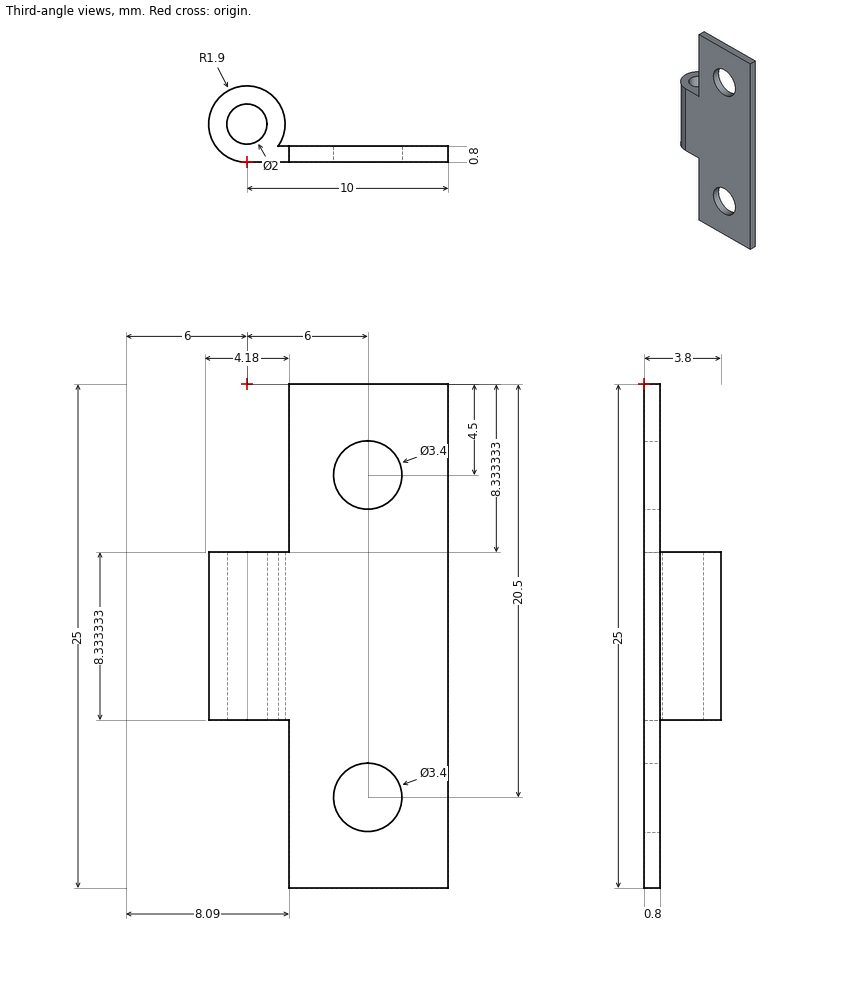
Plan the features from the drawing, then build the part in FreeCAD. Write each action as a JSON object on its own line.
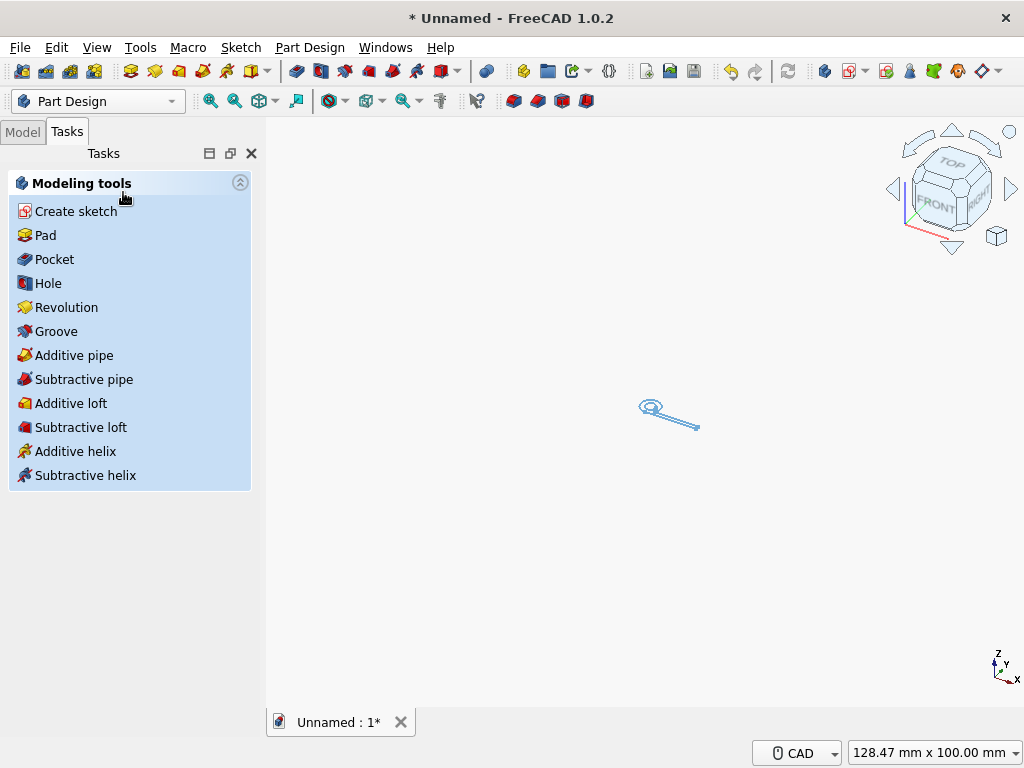
{"action": "left_click", "coordinate": [132, 72]}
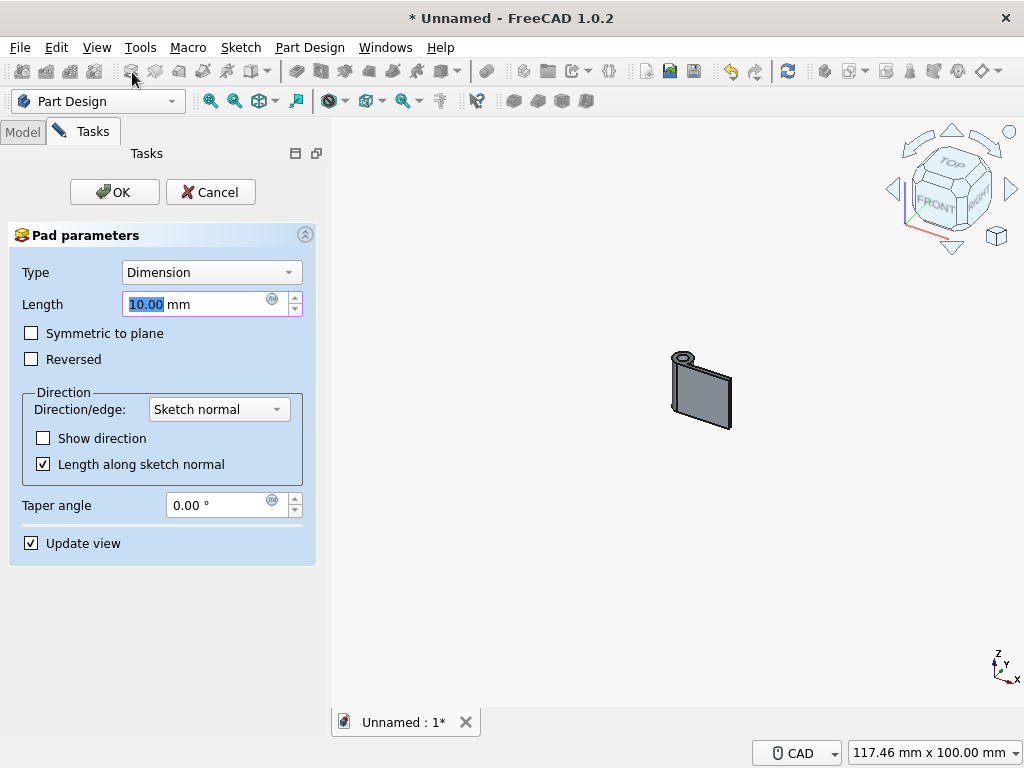
{"action": "type", "text": "25"}
{"action": "key", "text": "Tab"}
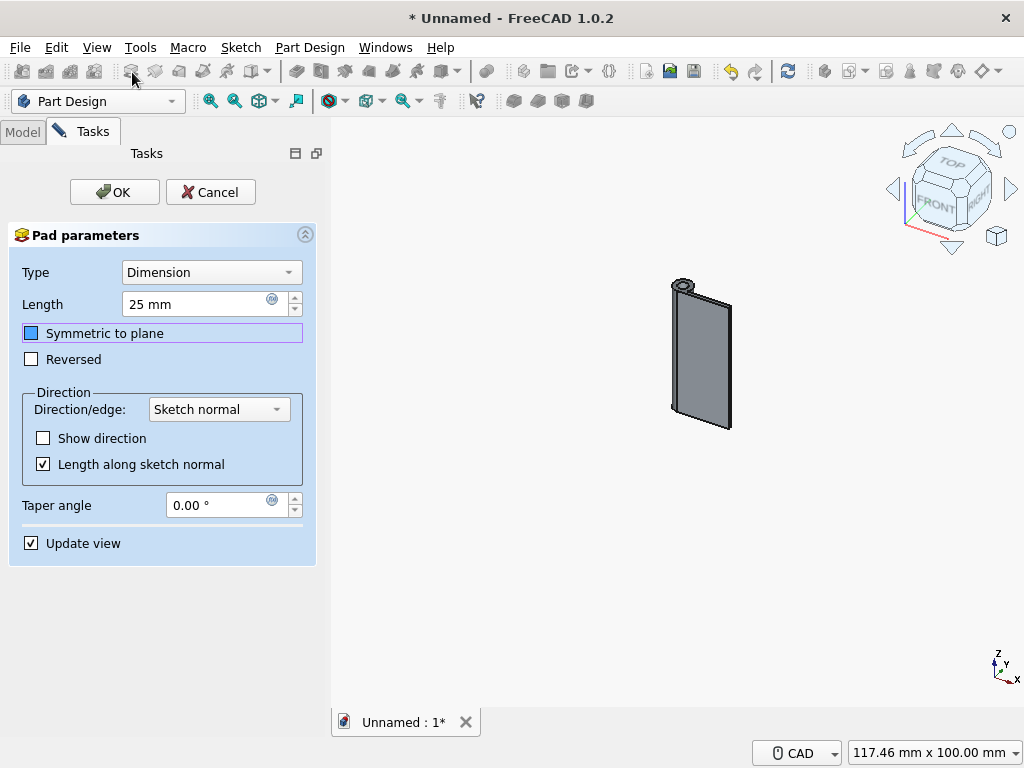
{"action": "left_click", "coordinate": [30, 359]}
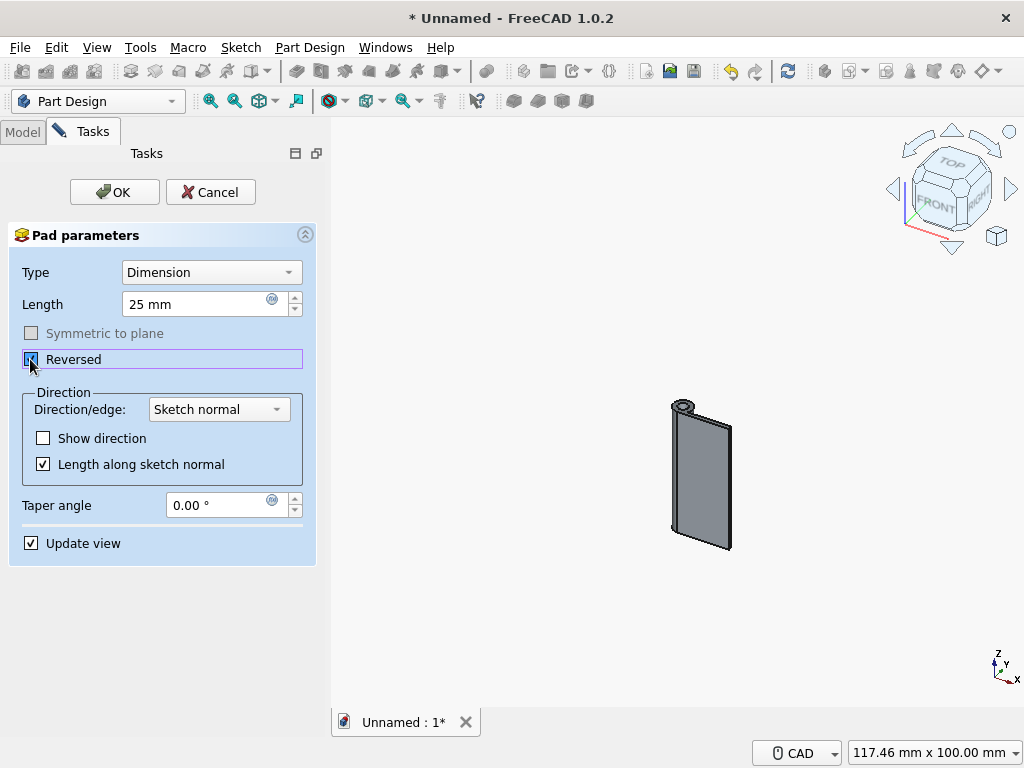
{"action": "left_click", "coordinate": [115, 192]}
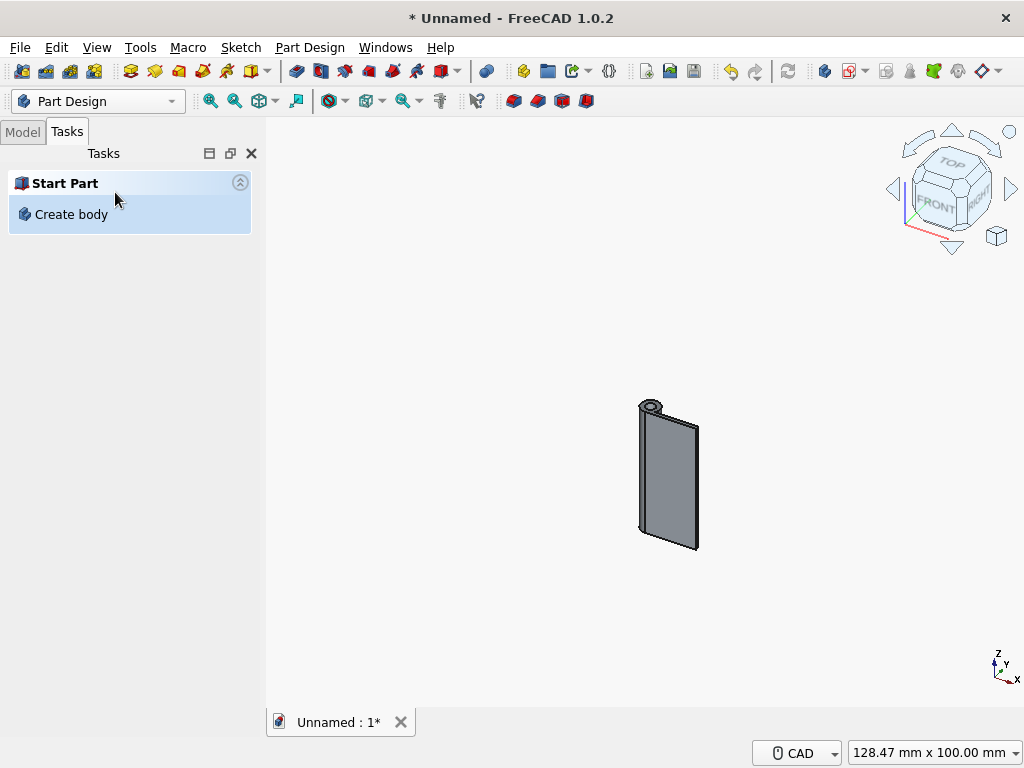
{"action": "key", "text": "v f"}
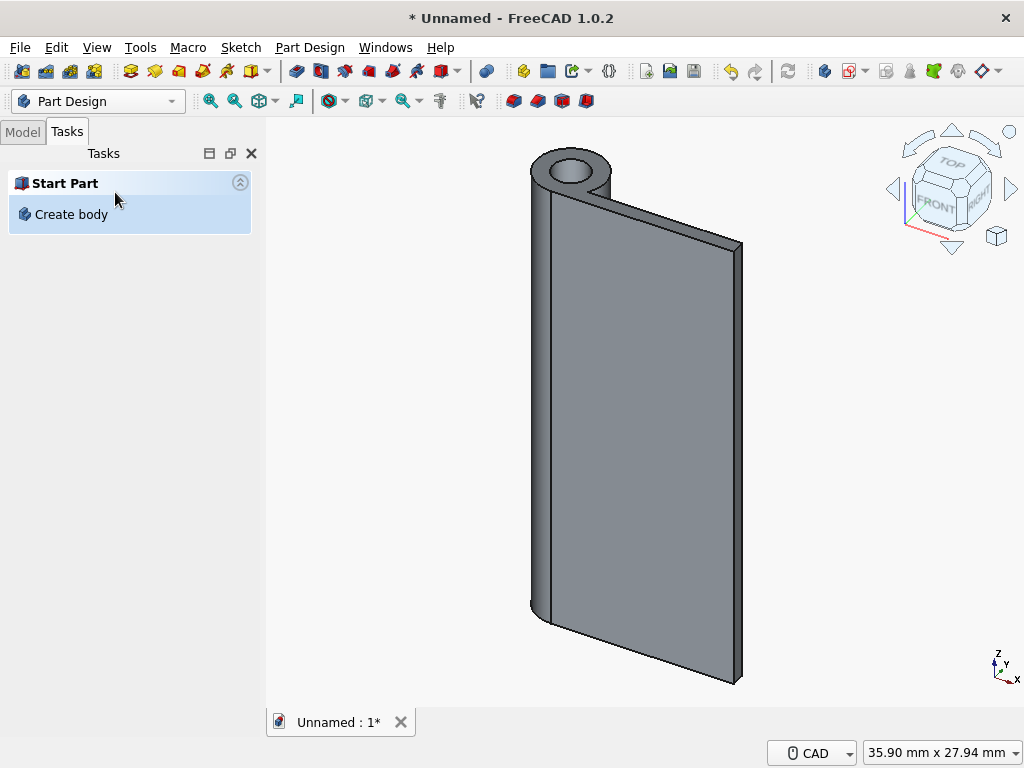
{"action": "left_click", "coordinate": [642, 313]}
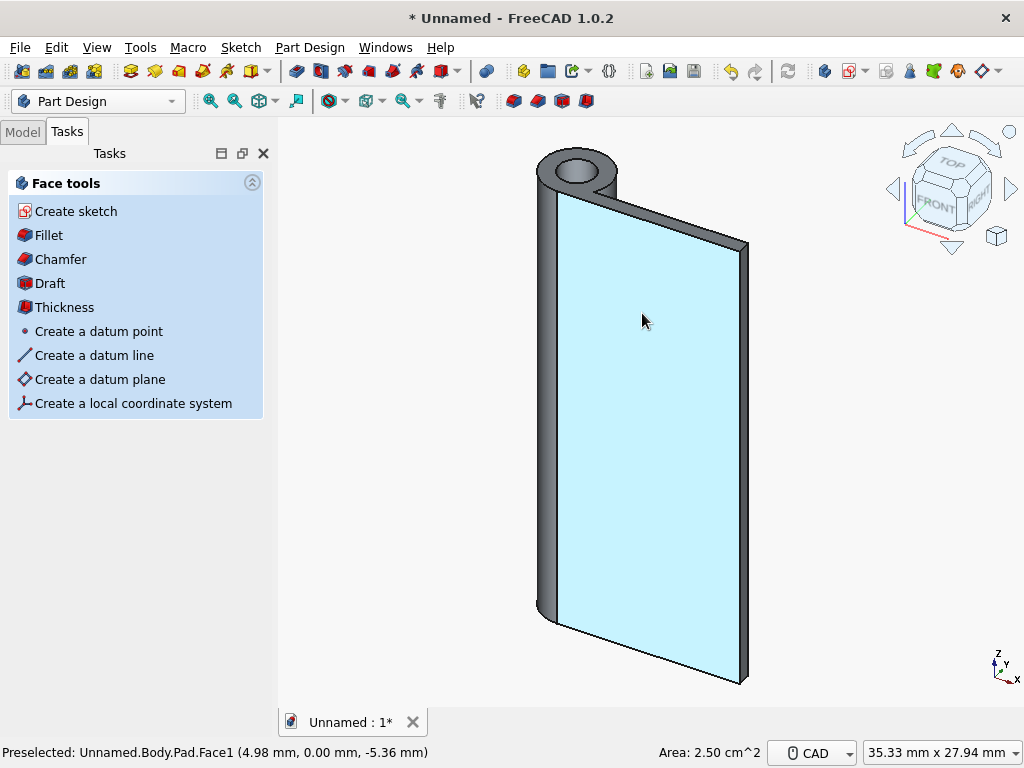
{"action": "left_click", "coordinate": [850, 72]}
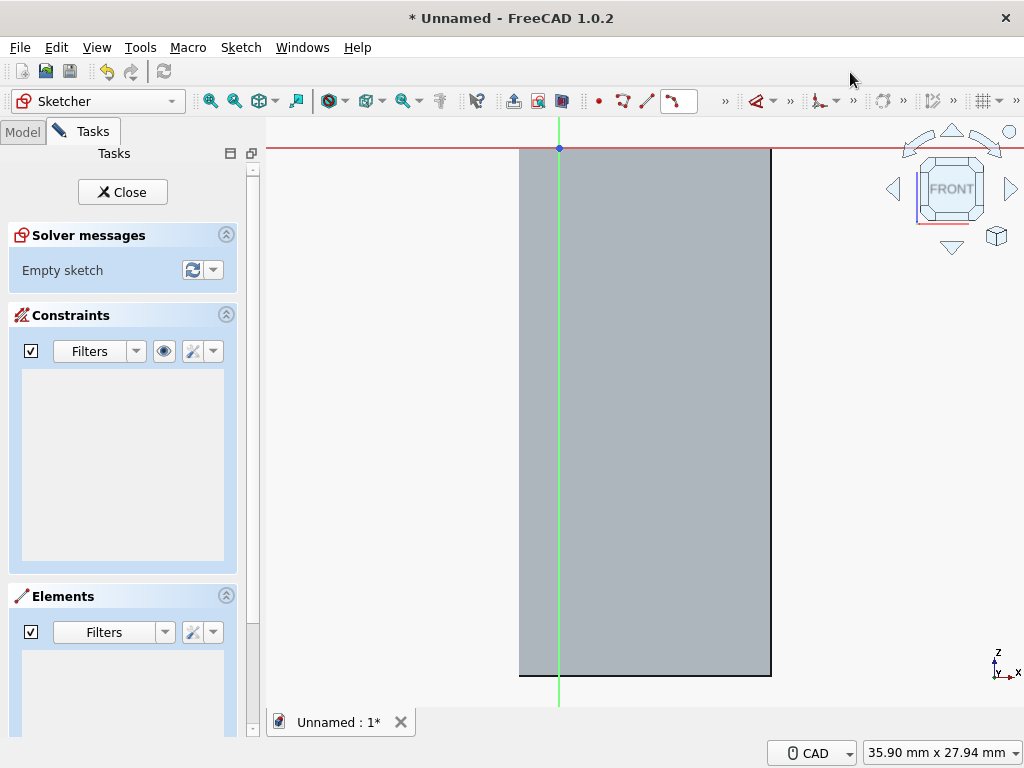
{"action": "scroll", "coordinate": [695, 412], "scroll_direction": "down", "scroll_amount": 2}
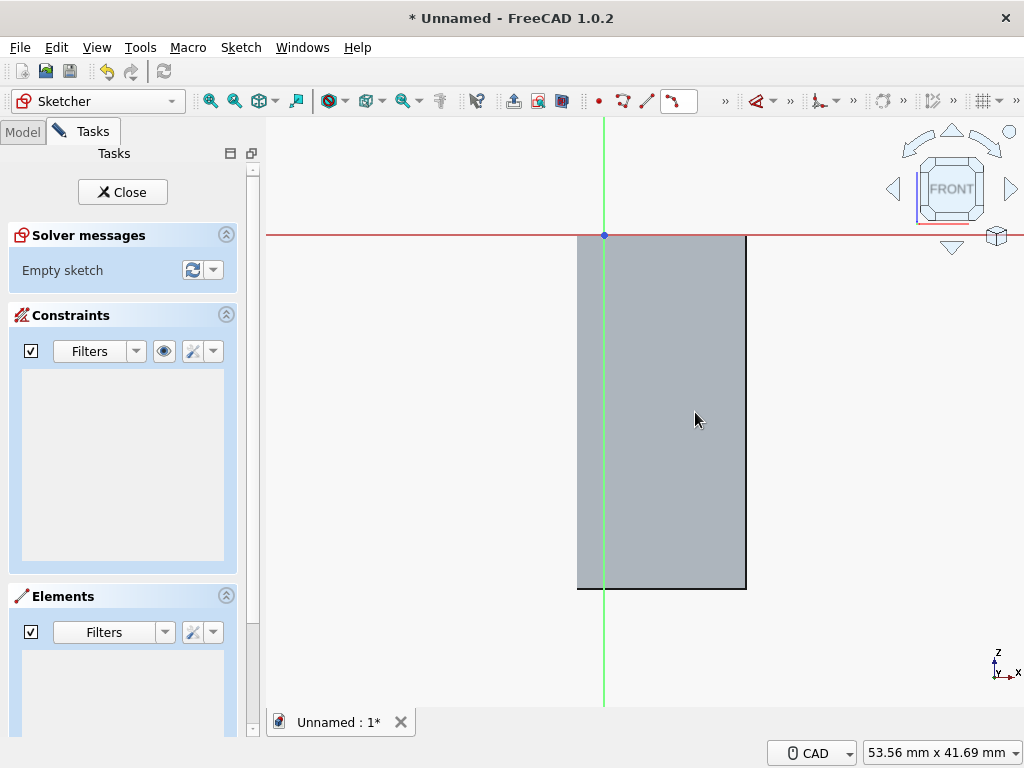
{"action": "left_click", "coordinate": [624, 102]}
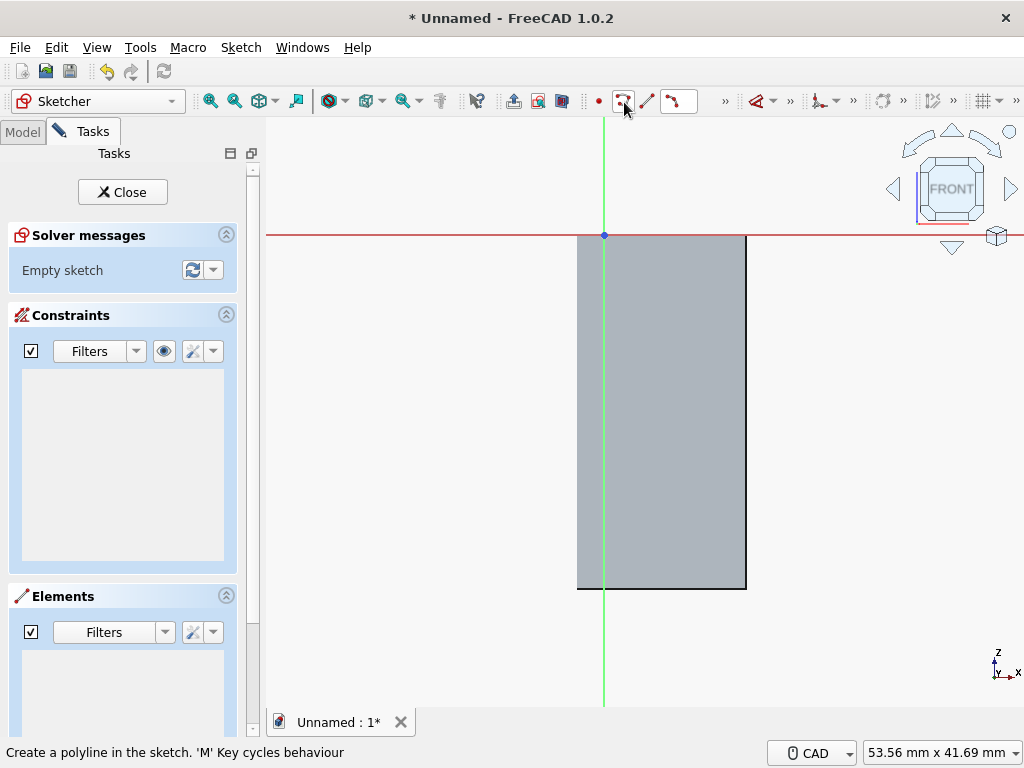
{"action": "left_click", "coordinate": [634, 235]}
{"action": "left_click", "coordinate": [634, 353]}
{"action": "left_click", "coordinate": [575, 353]}
{"action": "left_click", "coordinate": [575, 471]}
{"action": "left_click", "coordinate": [634, 471]}
{"action": "left_click", "coordinate": [634, 589]}
{"action": "left_click", "coordinate": [519, 589]}
{"action": "left_click", "coordinate": [519, 244]}
{"action": "left_click", "coordinate": [634, 235]}
{"action": "key", "text": "Escape"}
{"action": "key", "text": "Escape"}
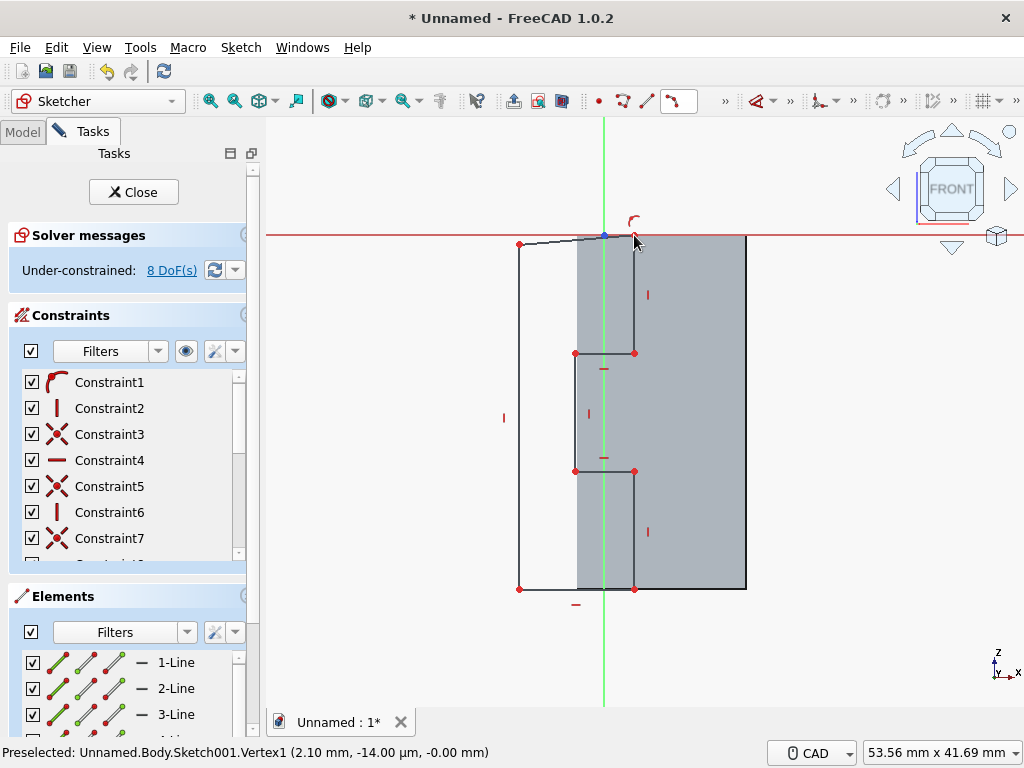
{"action": "left_click", "coordinate": [588, 239]}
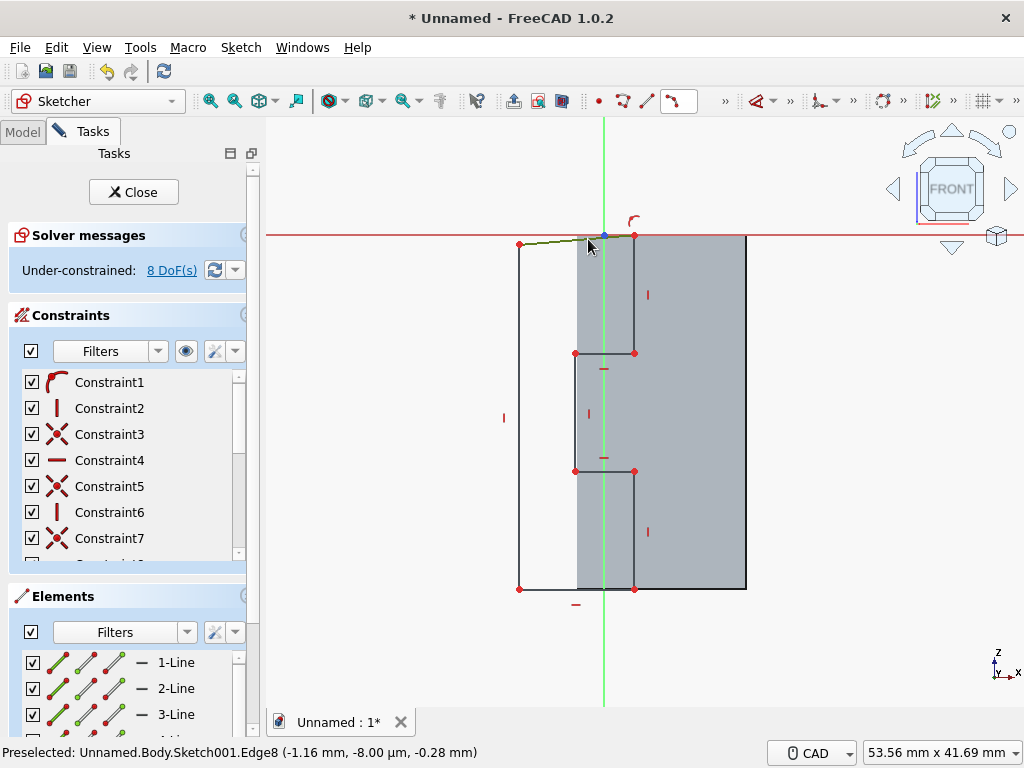
{"action": "key", "text": "h"}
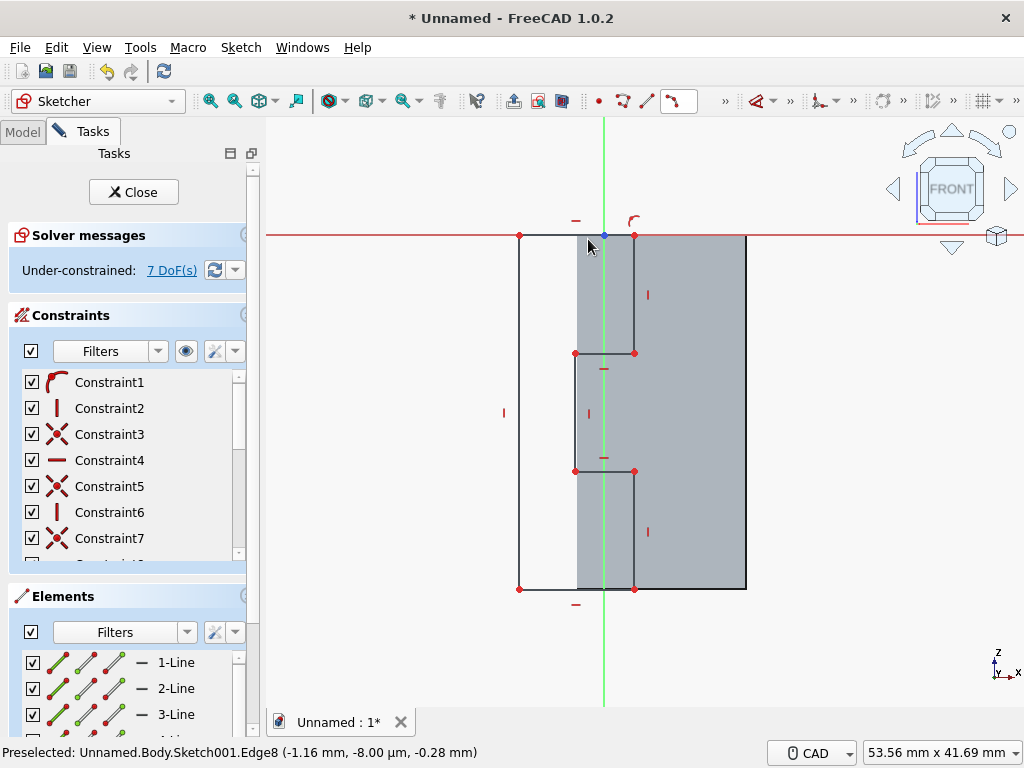
{"action": "left_click", "coordinate": [756, 102]}